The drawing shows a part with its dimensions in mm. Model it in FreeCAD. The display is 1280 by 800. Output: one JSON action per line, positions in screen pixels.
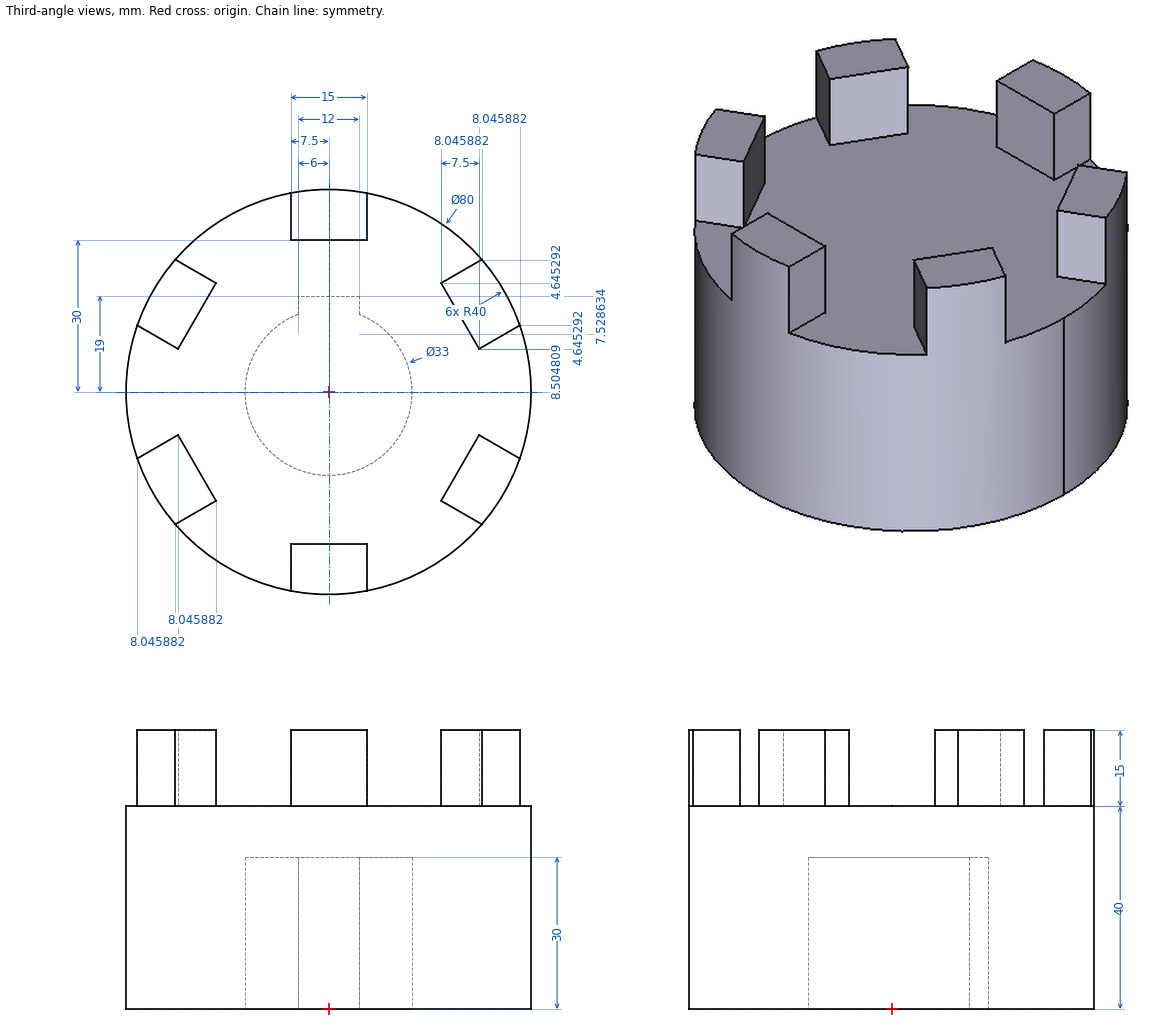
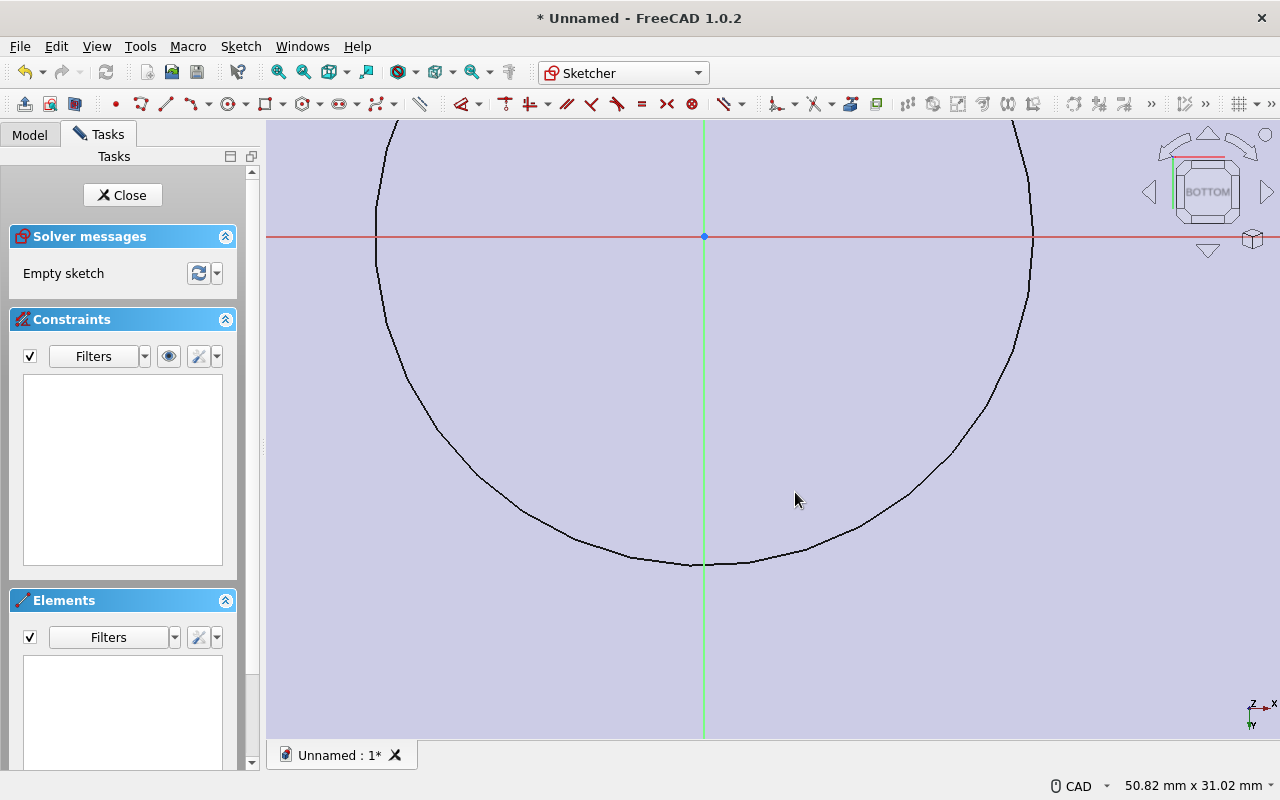
{"action": "left_click", "coordinate": [264, 104]}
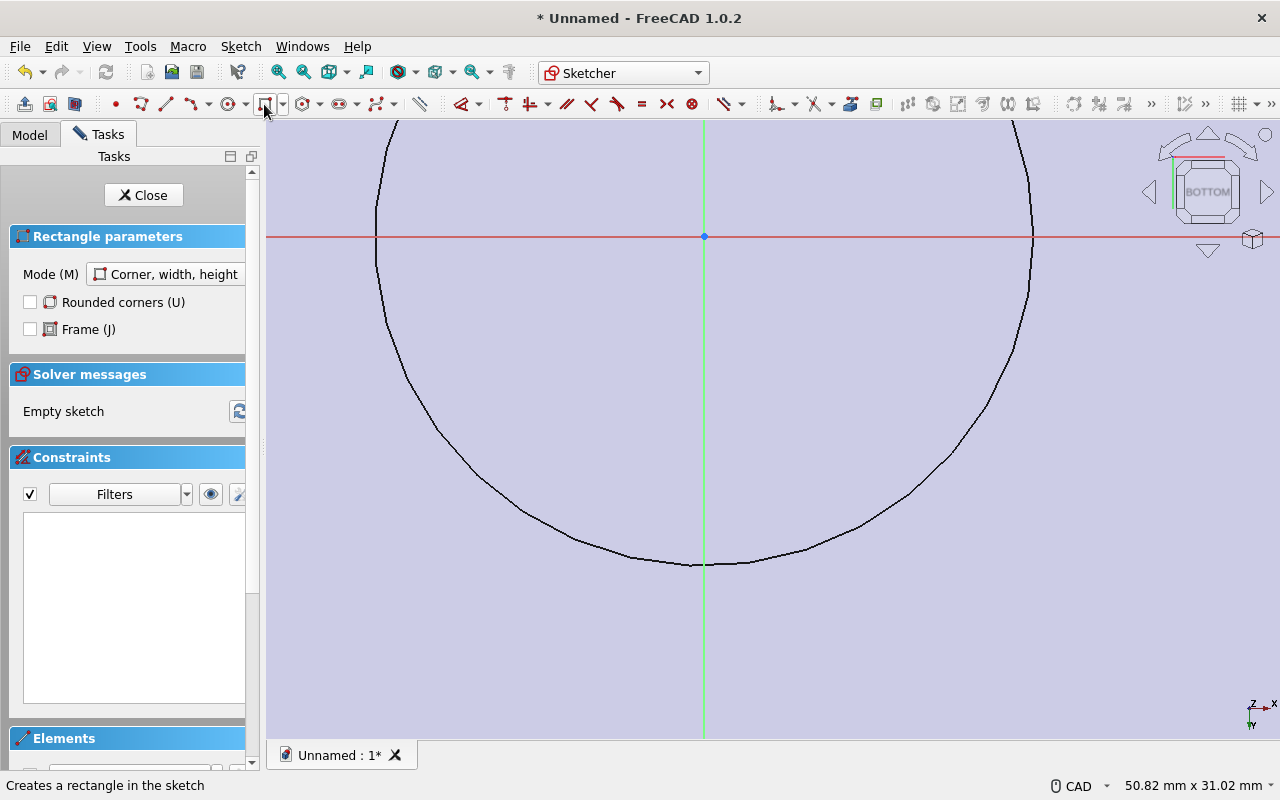
{"action": "left_click", "coordinate": [584, 466]}
{"action": "mouse_move", "coordinate": [824, 616]}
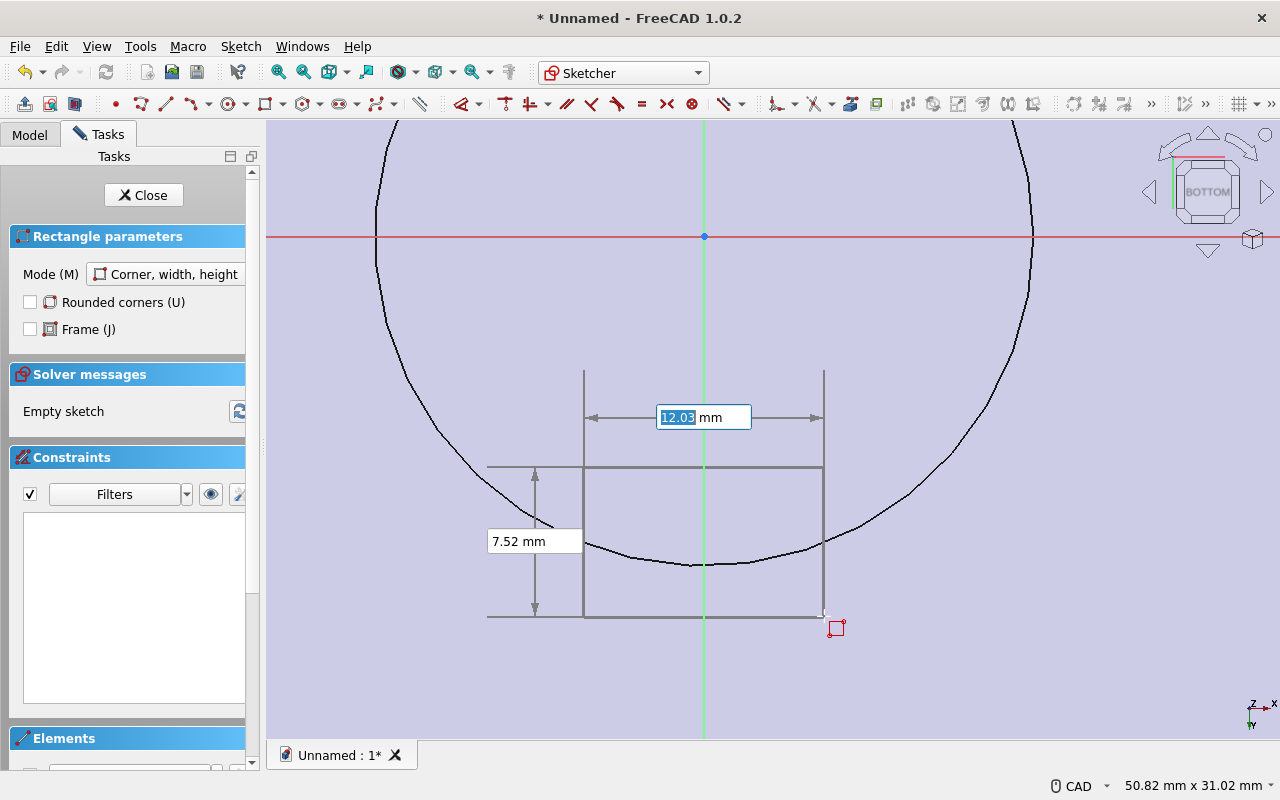
{"action": "type", "text": "12"}
{"action": "key", "text": "Tab"}
{"action": "type", "text": "7.528634"}
{"action": "key", "text": "Return"}
{"action": "key", "text": "Escape"}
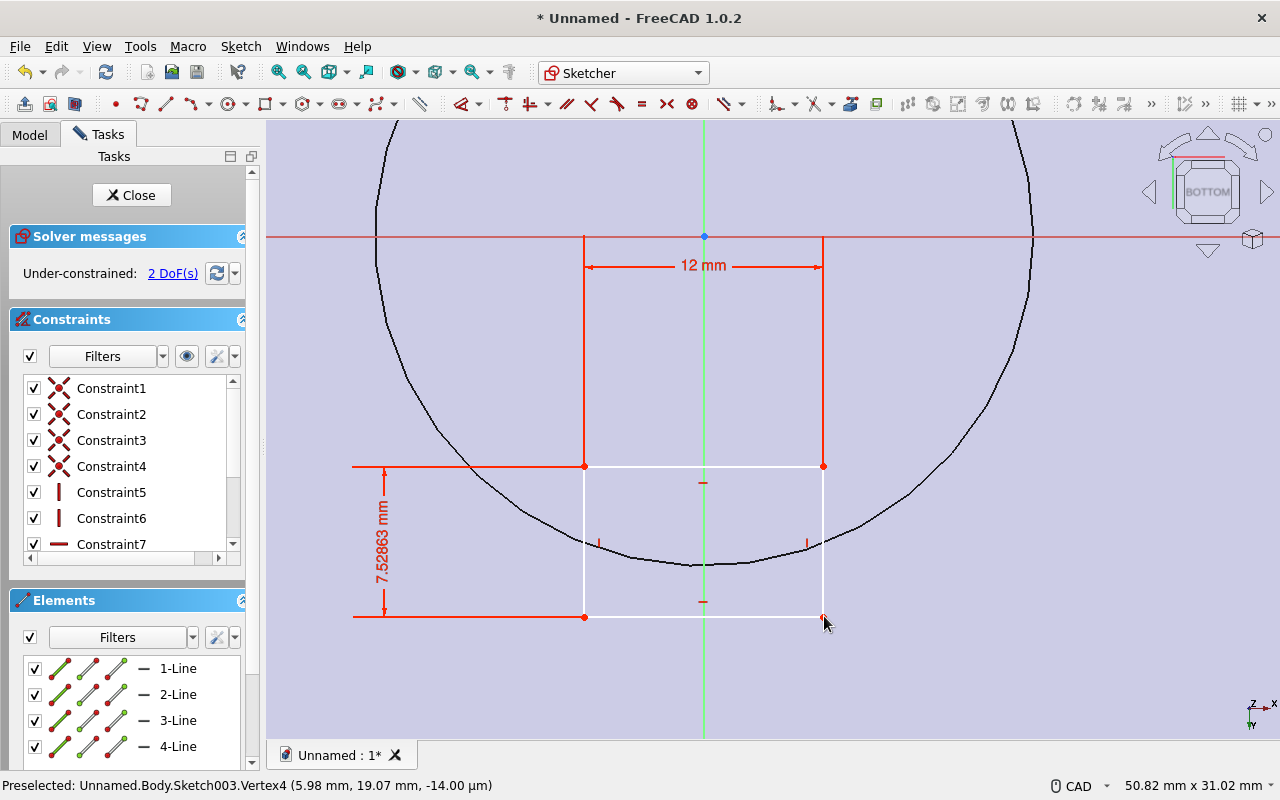
{"action": "key", "text": "d"}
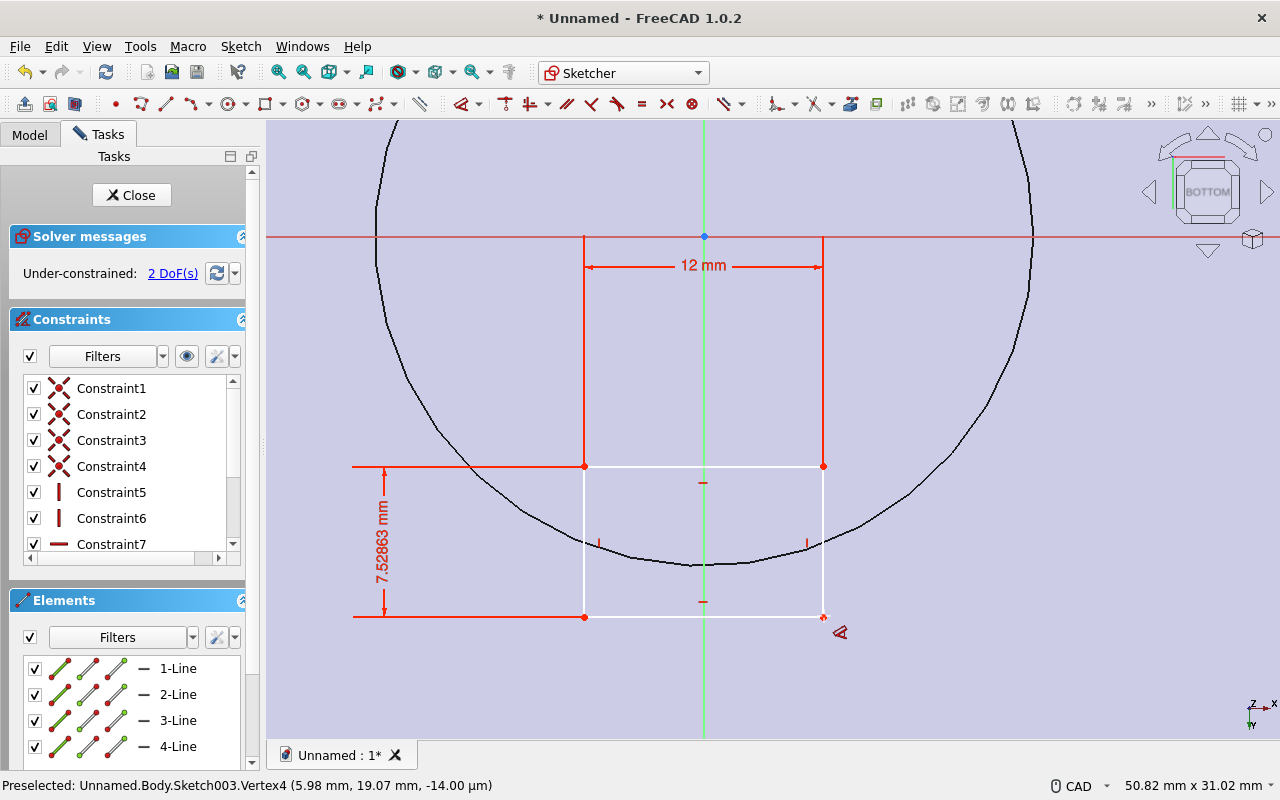
{"action": "left_click", "coordinate": [584, 467]}
{"action": "left_click", "coordinate": [644, 203]}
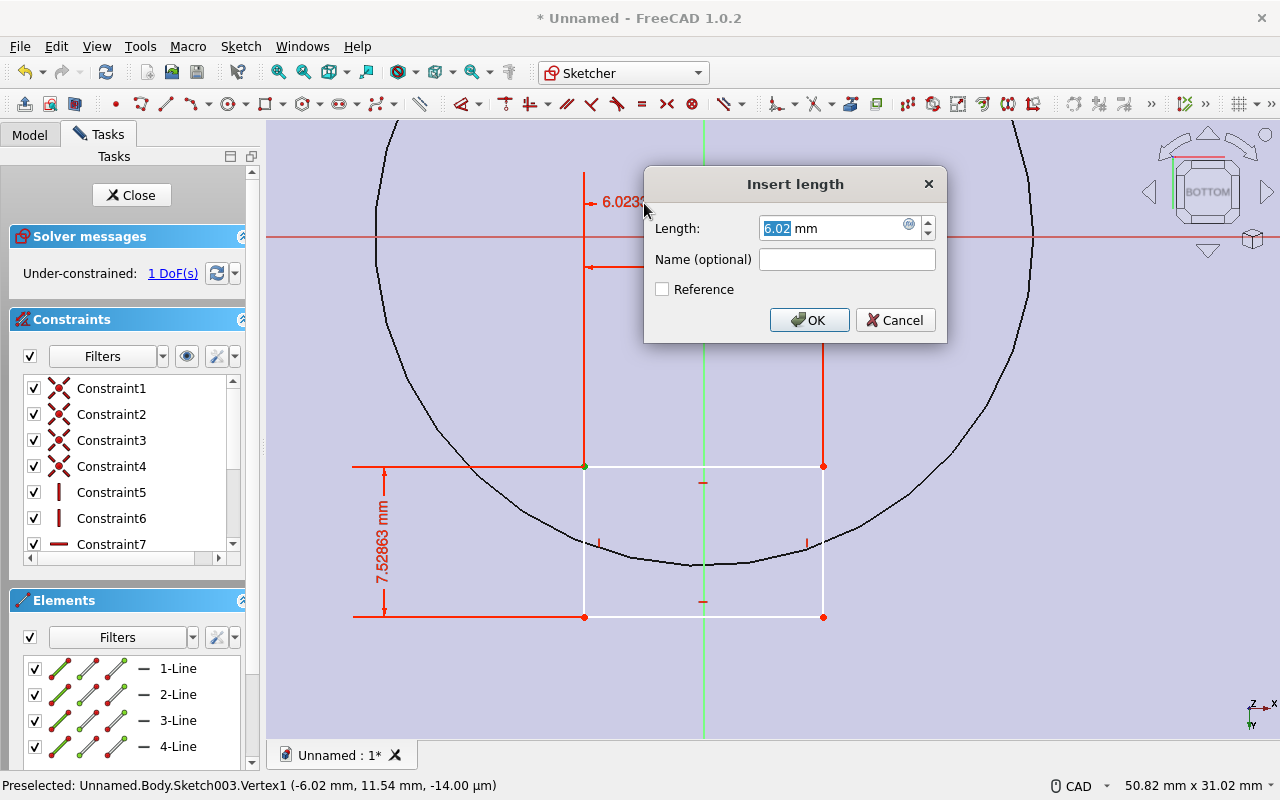
{"action": "type", "text": "6"}
{"action": "key", "text": "Return"}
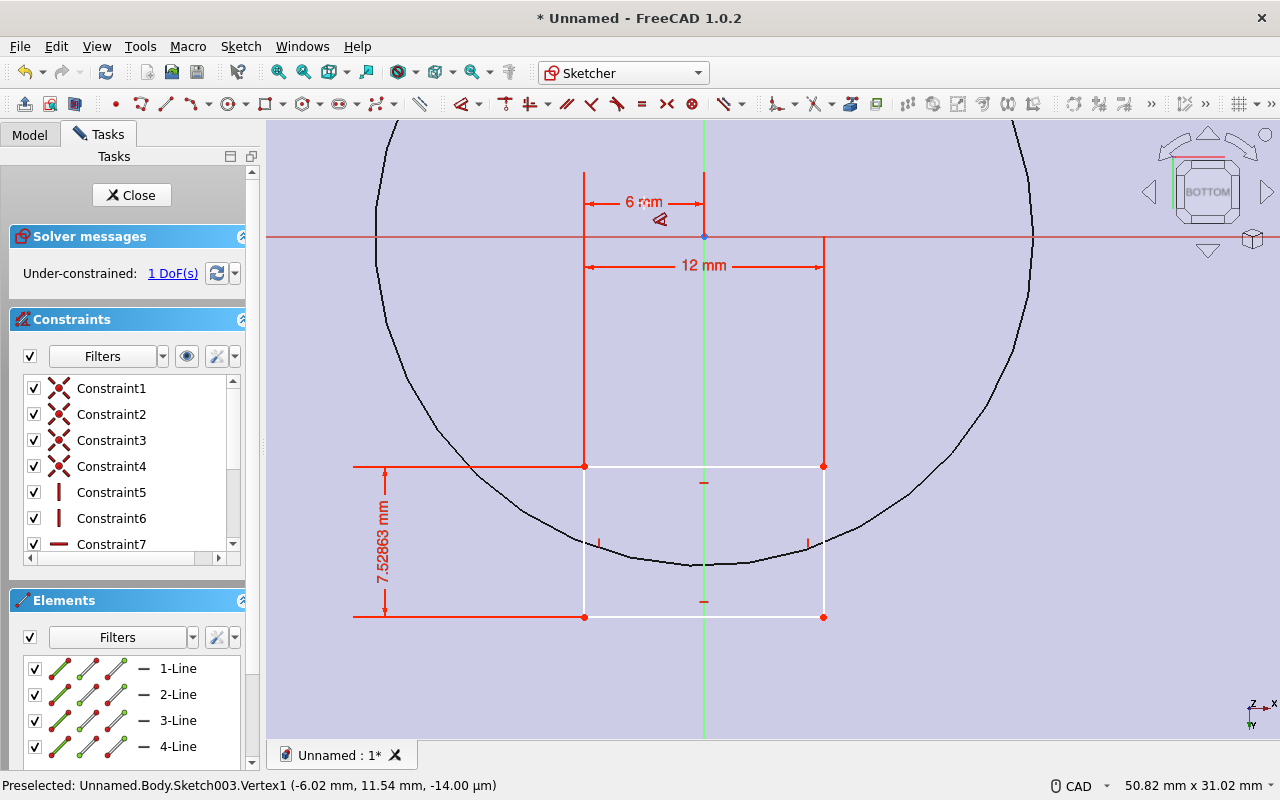
{"action": "left_click", "coordinate": [584, 617]}
{"action": "left_click", "coordinate": [550, 427]}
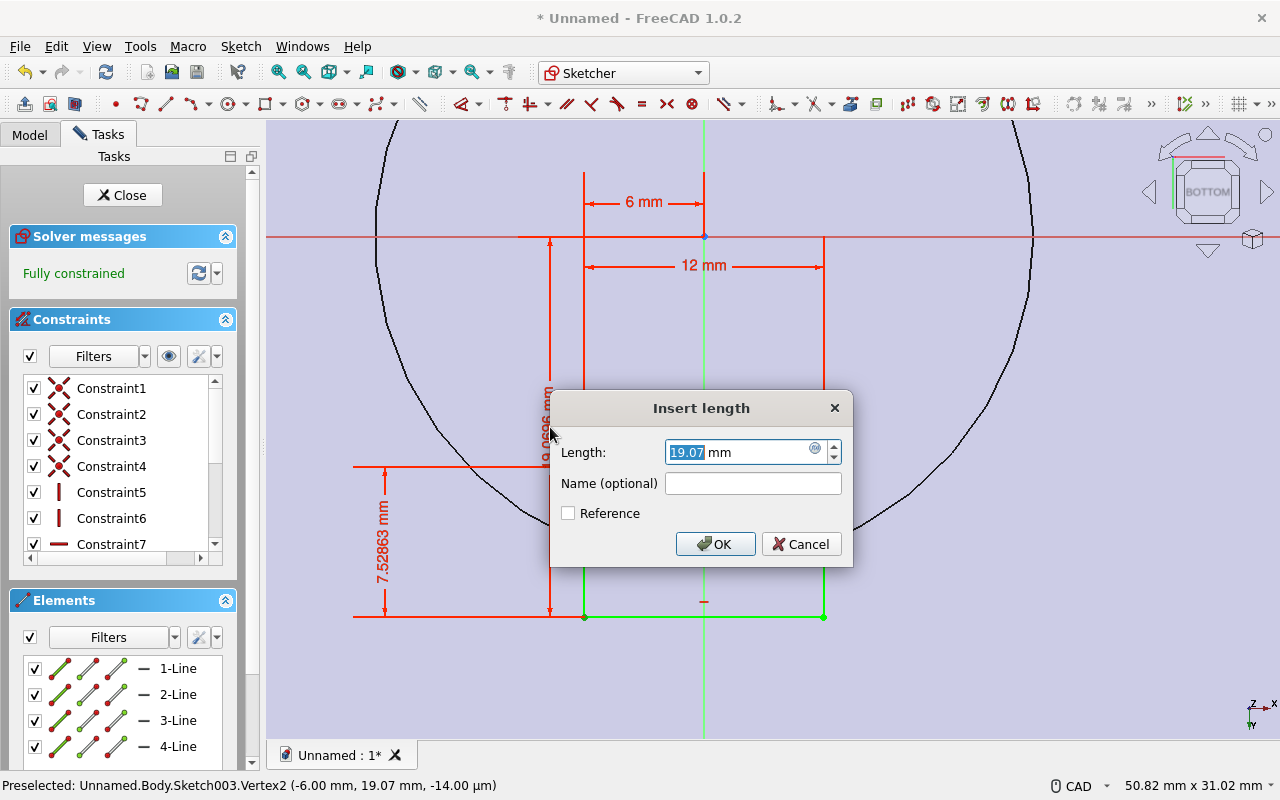
{"action": "type", "text": "19"}
{"action": "key", "text": "Return"}
{"action": "key", "text": "Escape"}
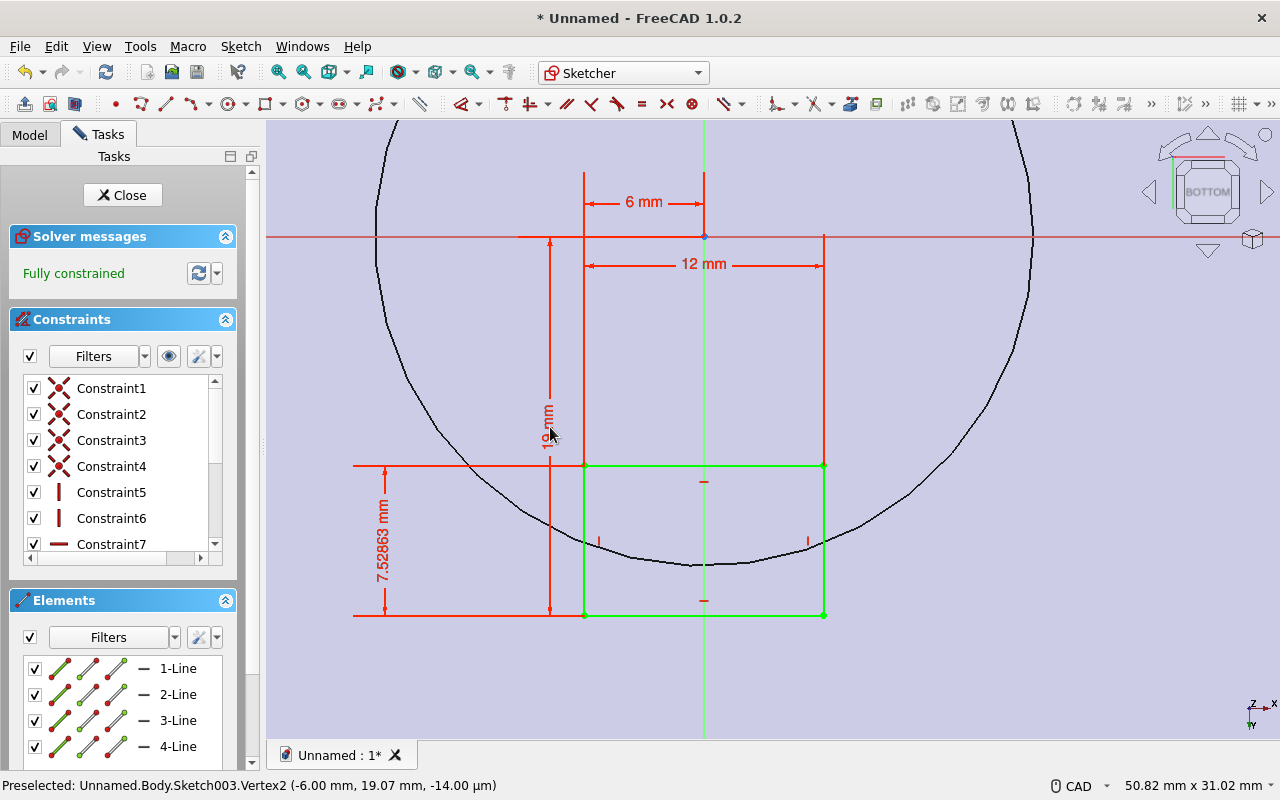
{"action": "left_click", "coordinate": [123, 195]}